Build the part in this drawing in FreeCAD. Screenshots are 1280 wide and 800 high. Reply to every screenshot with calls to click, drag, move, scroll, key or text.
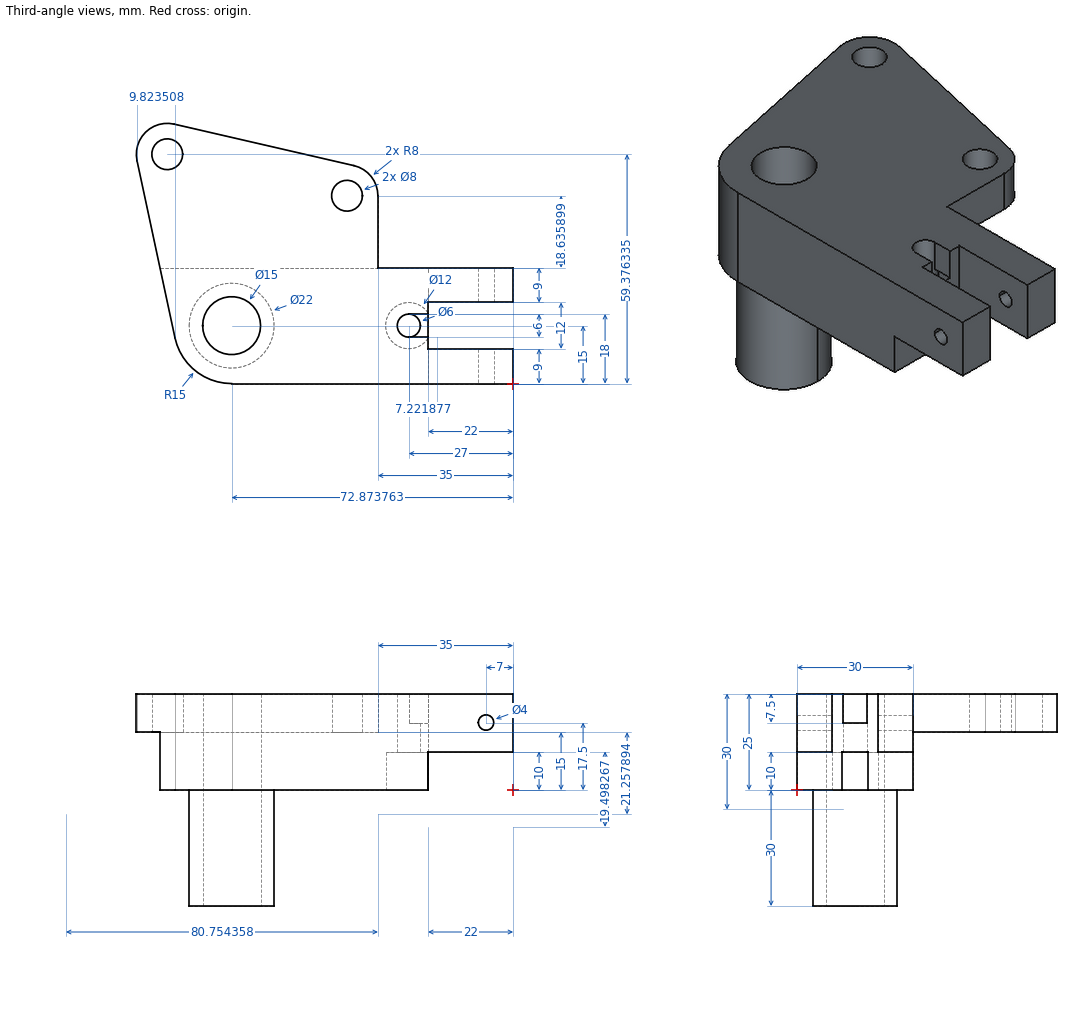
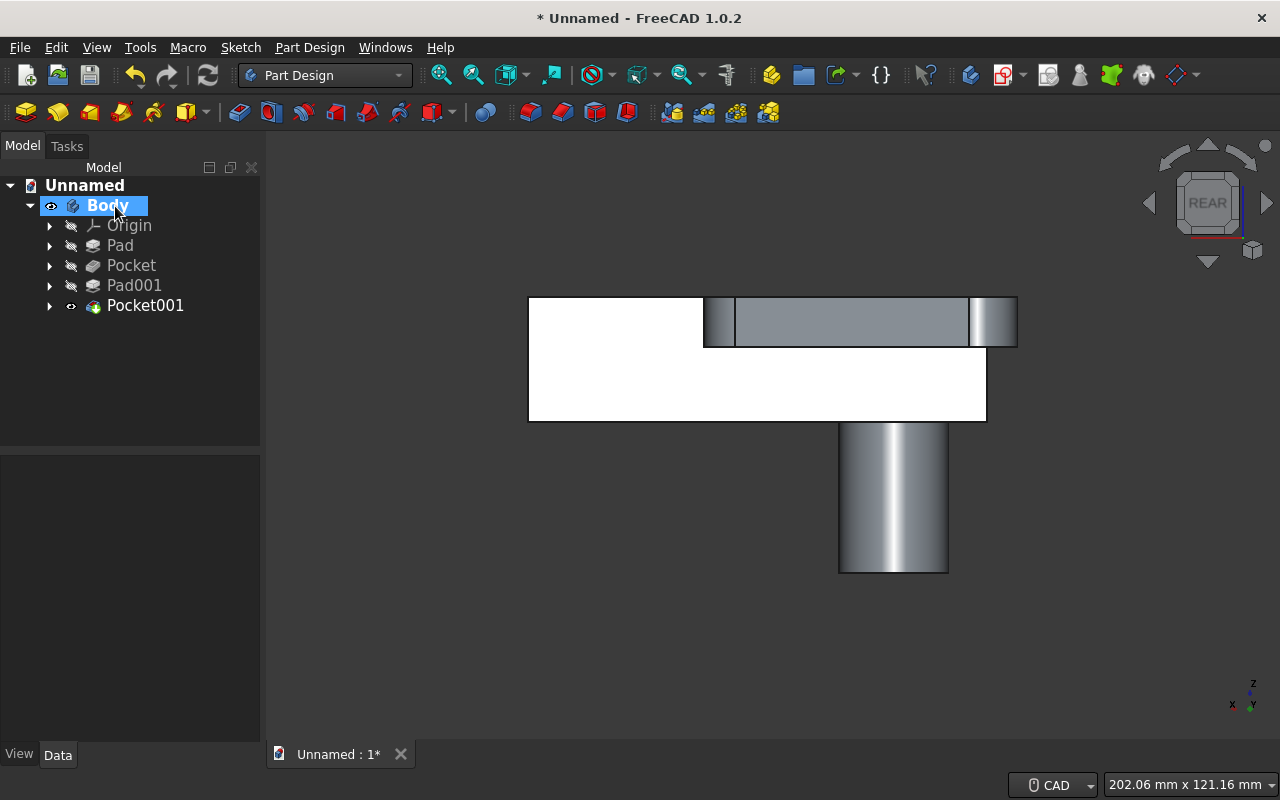
click(627, 359)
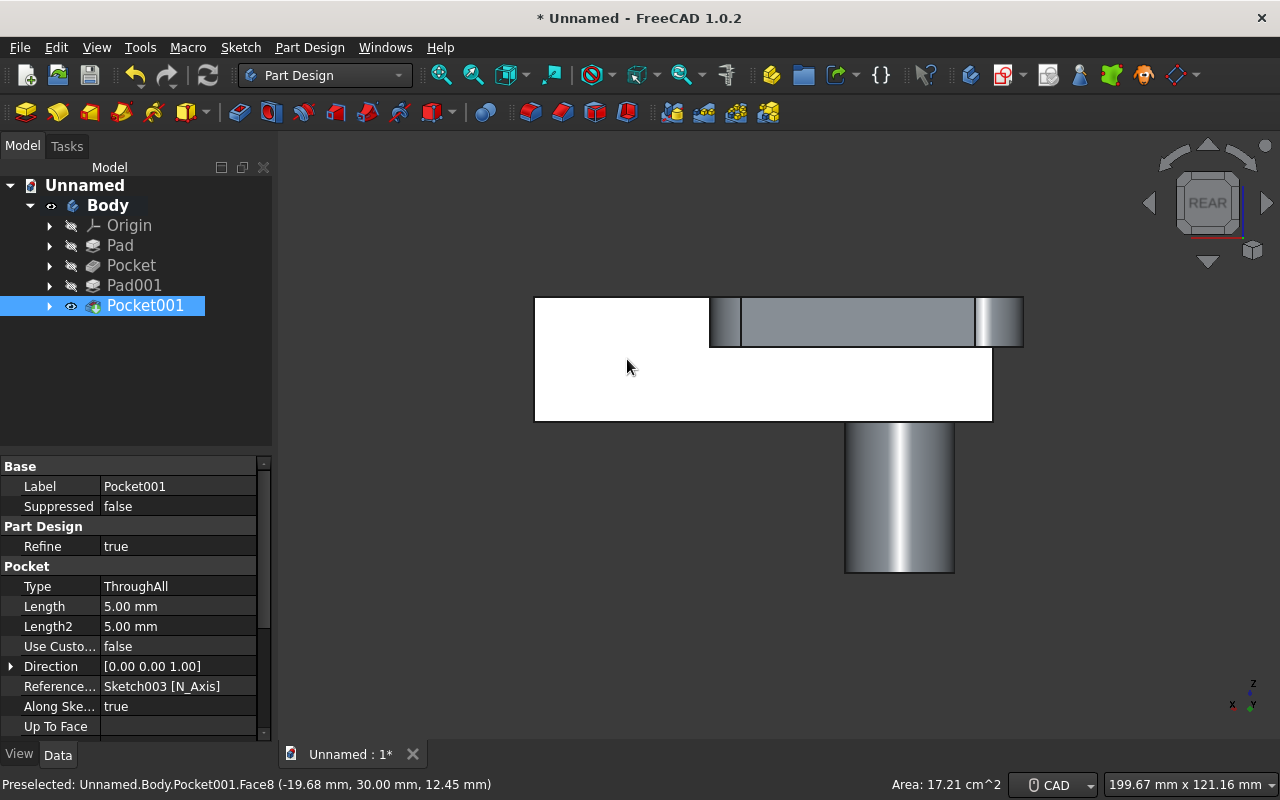
click(1004, 76)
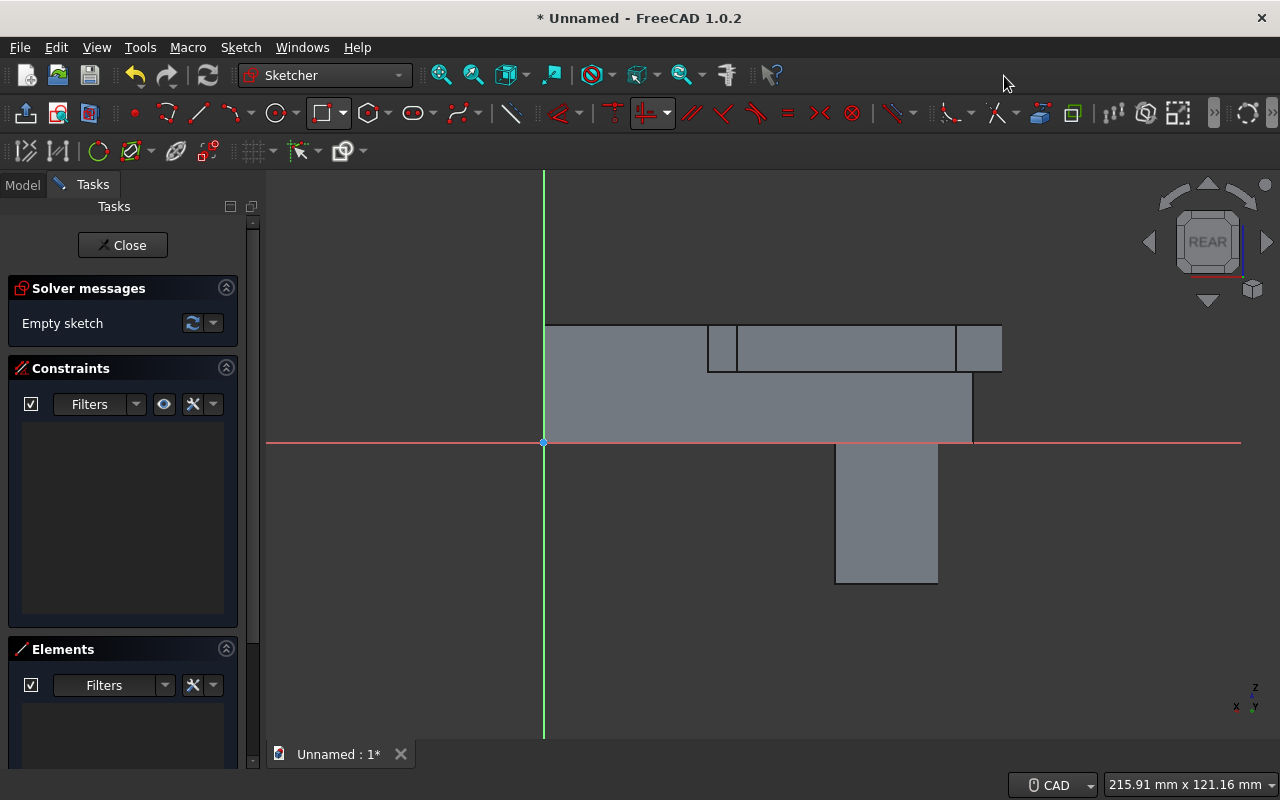
click(90, 114)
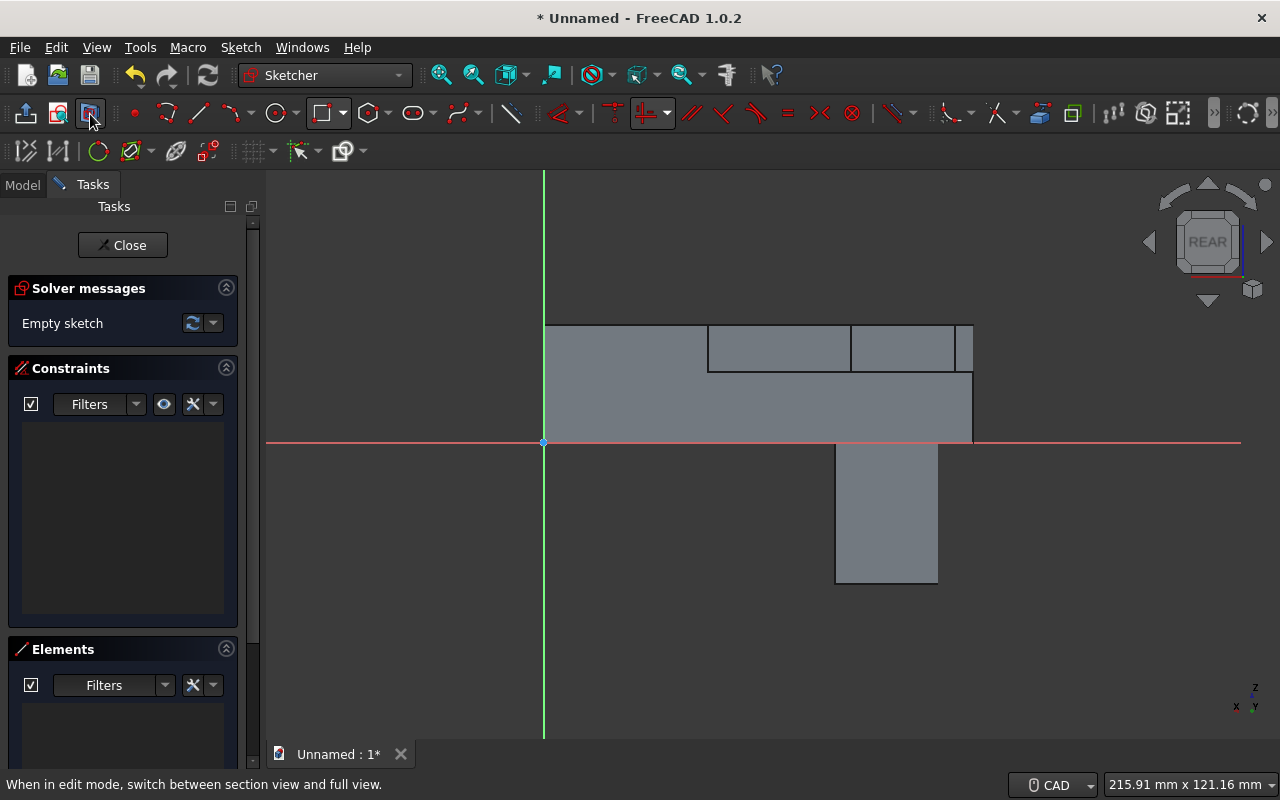
scroll(560, 437, up, 7)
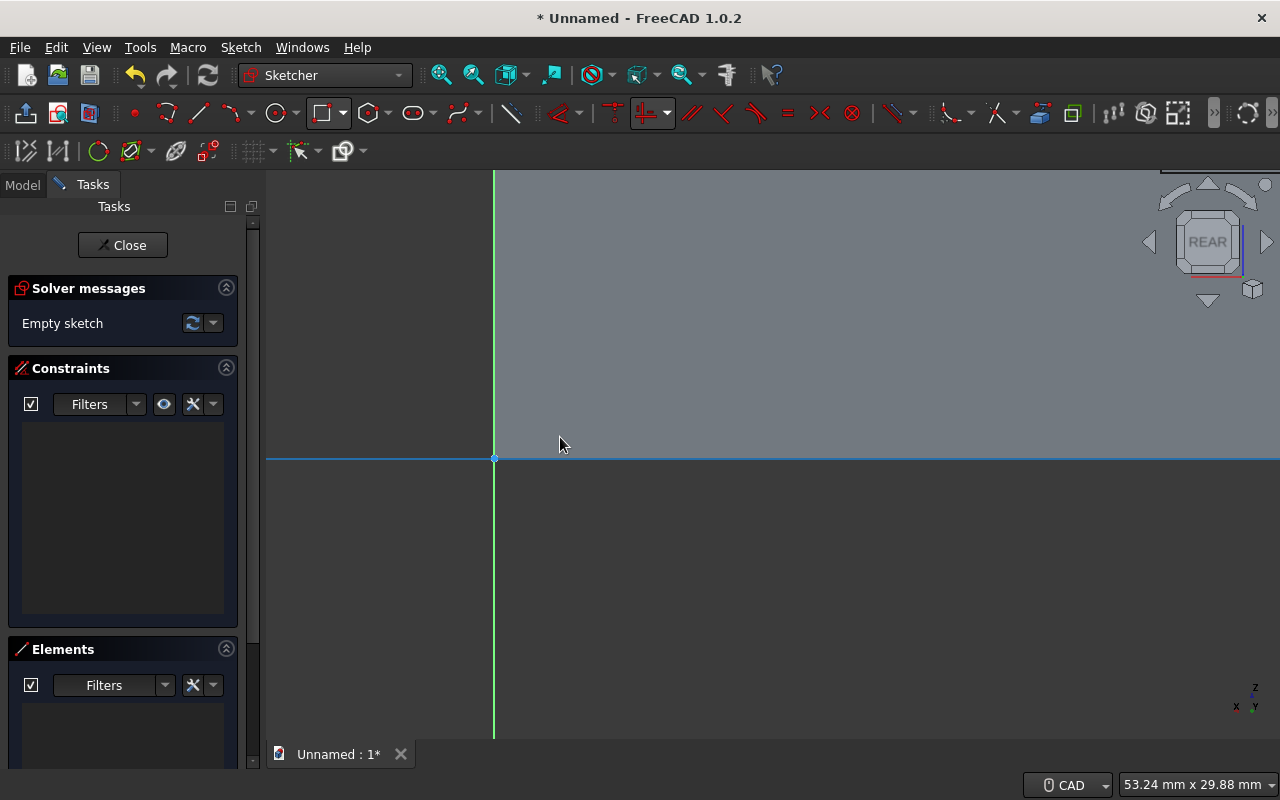
key(g)
key(r)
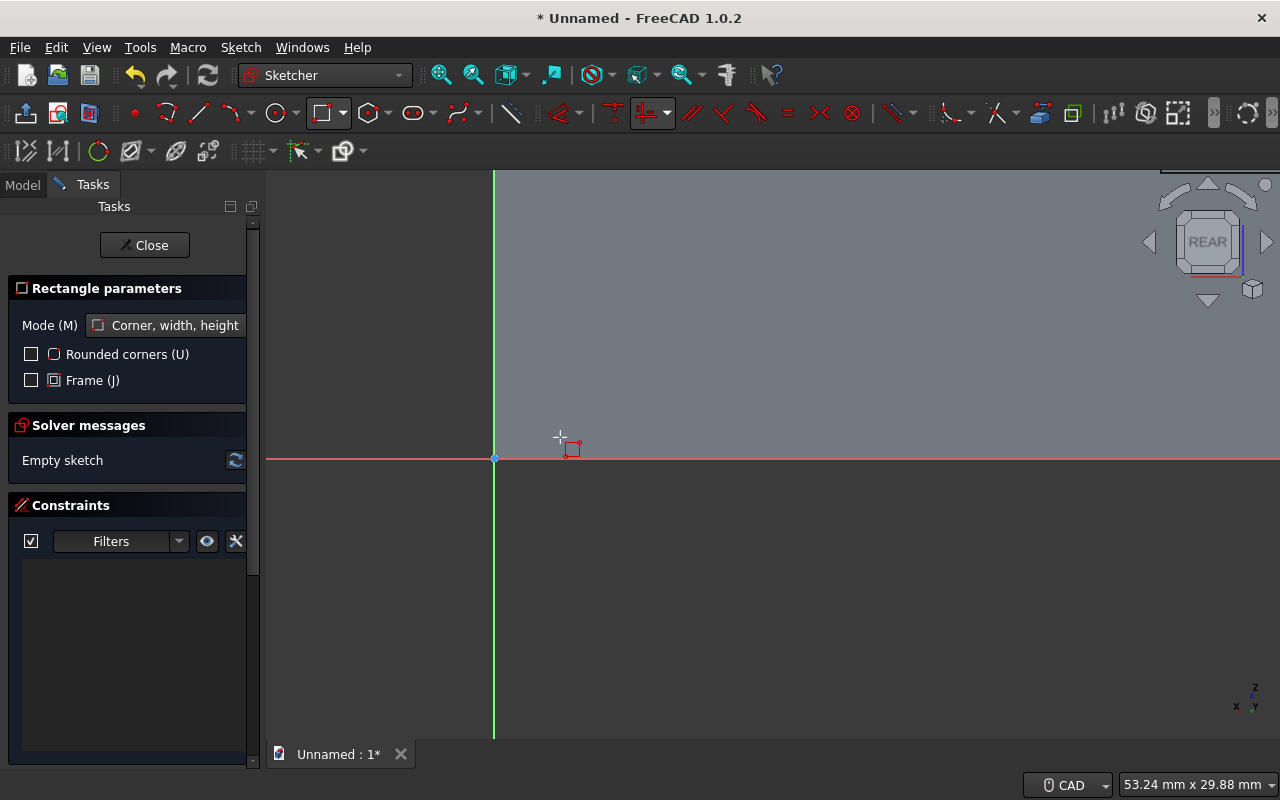
click(494, 268)
click(913, 640)
key(Escape)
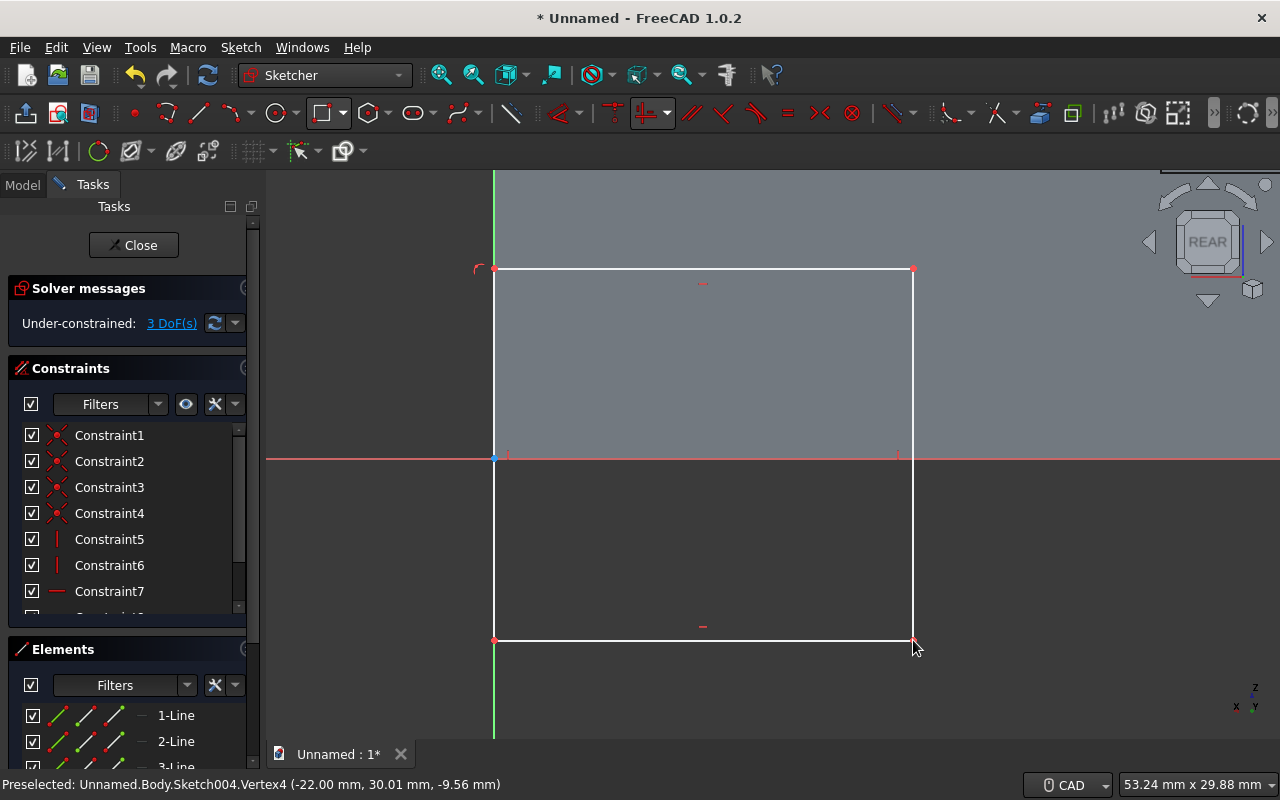
click(558, 114)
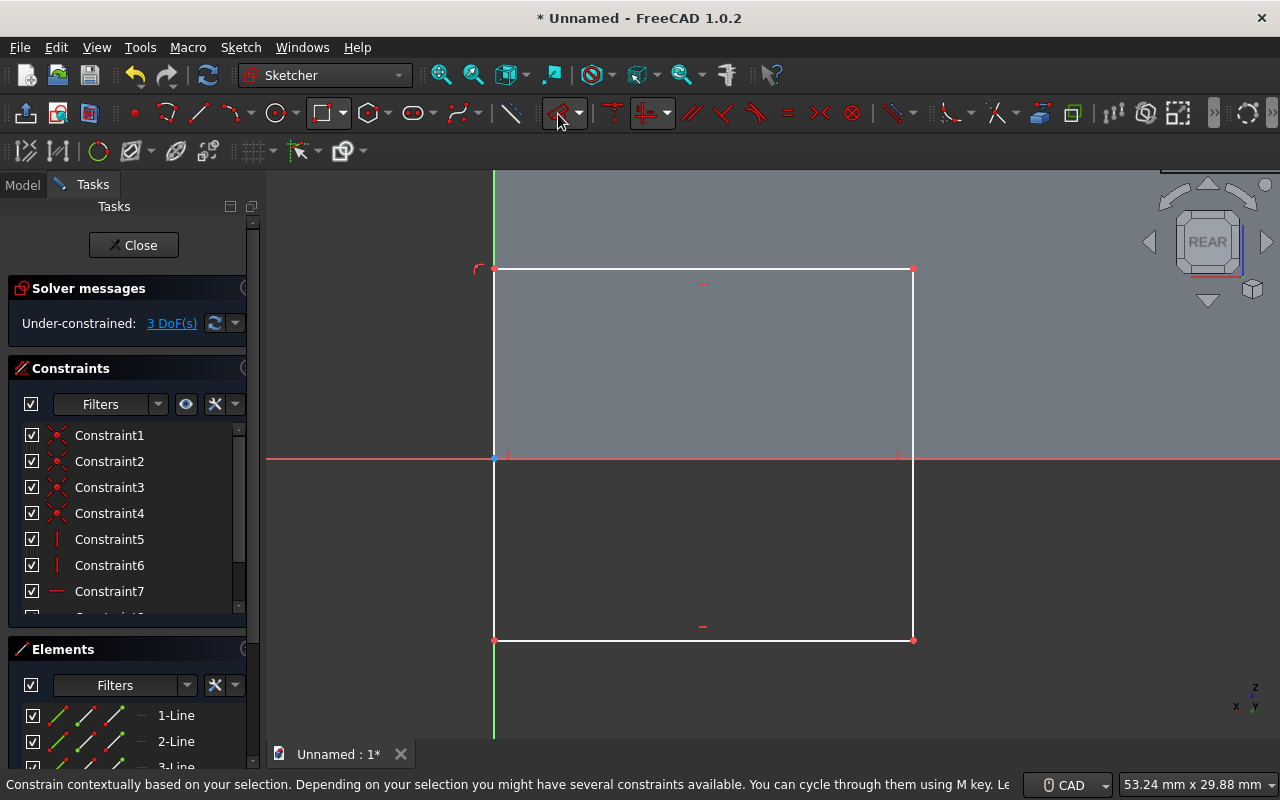
click(620, 641)
click(704, 675)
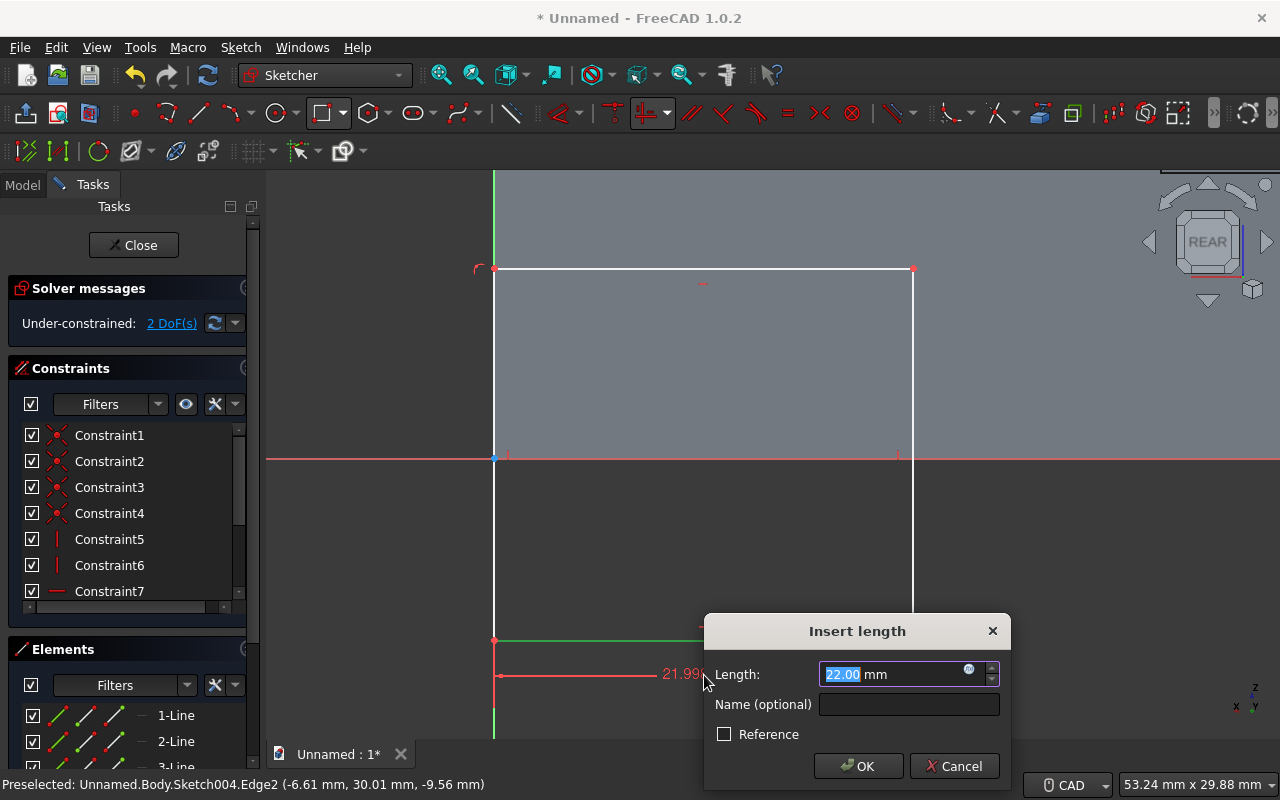
text(22)
key(Return)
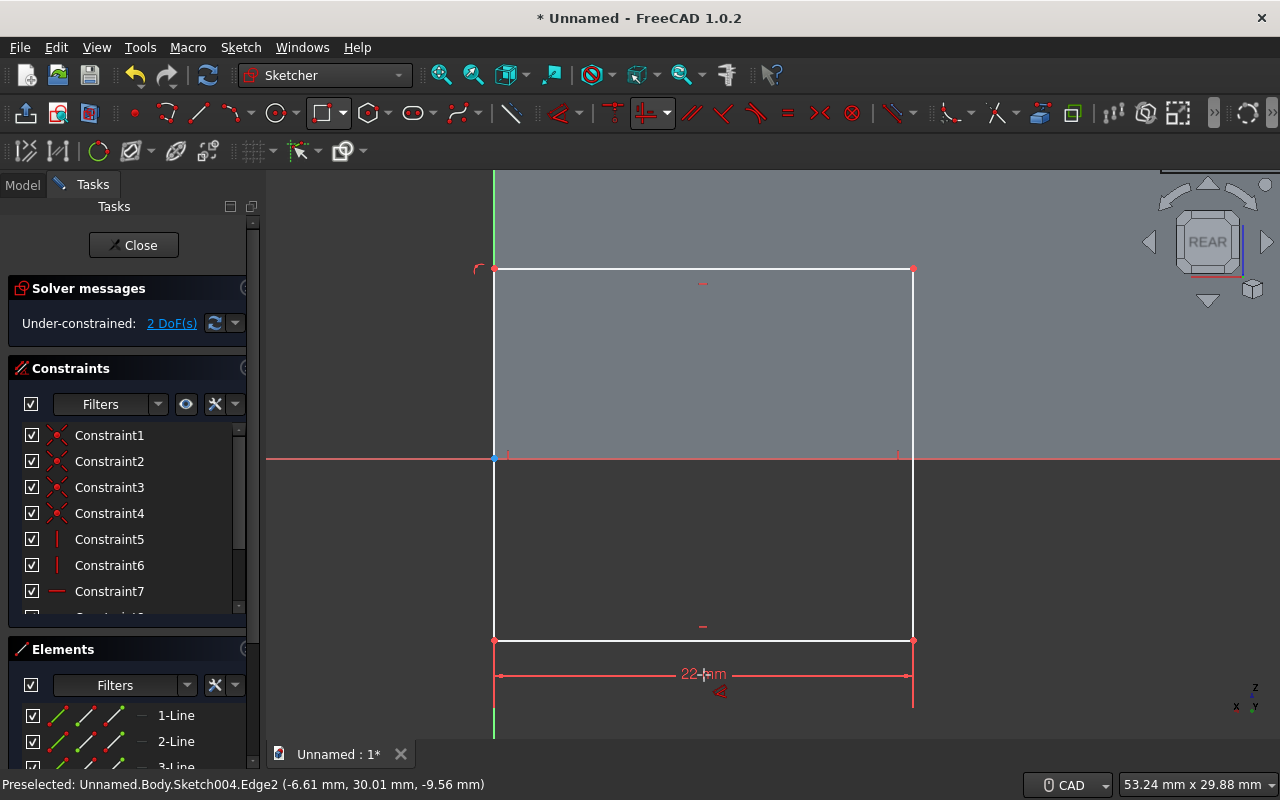
click(494, 269)
click(460, 364)